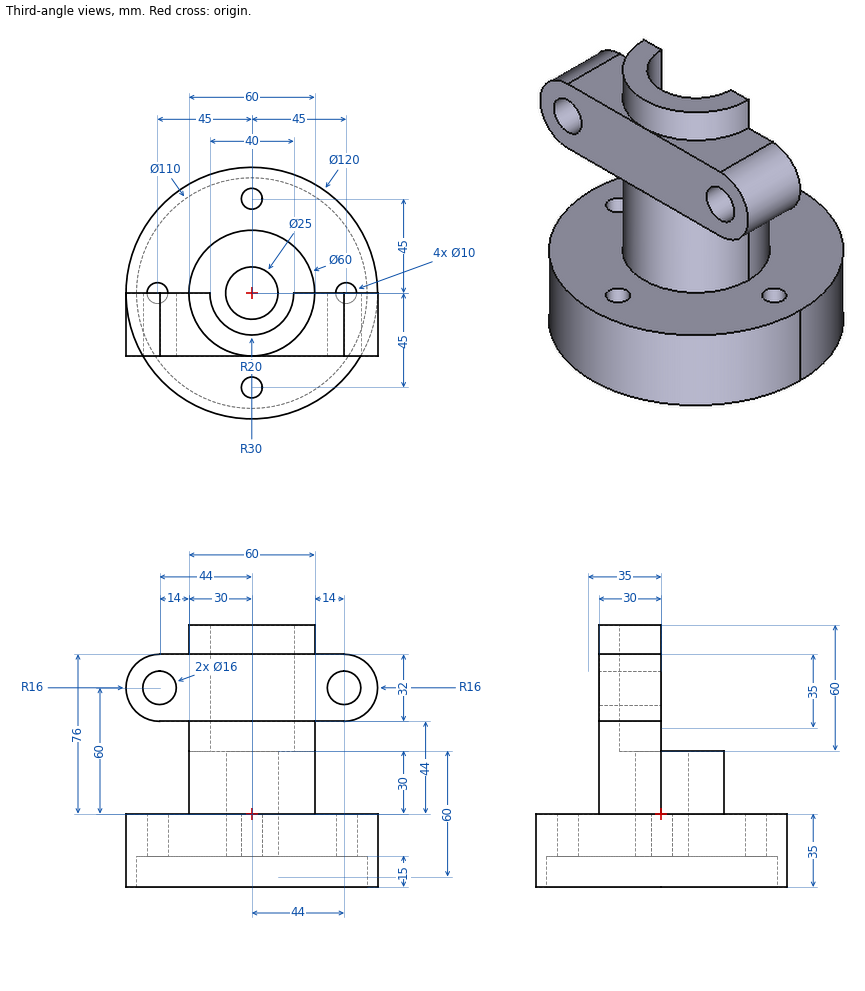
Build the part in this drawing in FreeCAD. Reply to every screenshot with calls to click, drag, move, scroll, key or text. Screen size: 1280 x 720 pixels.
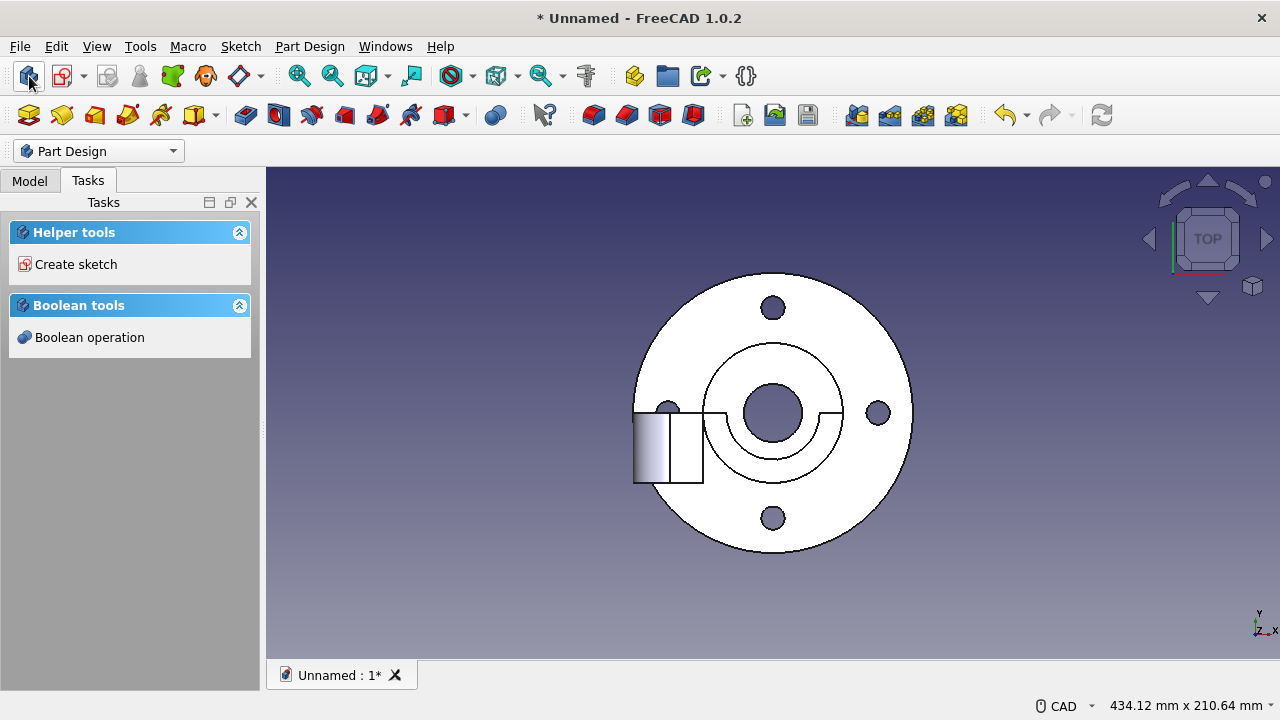
click(306, 619)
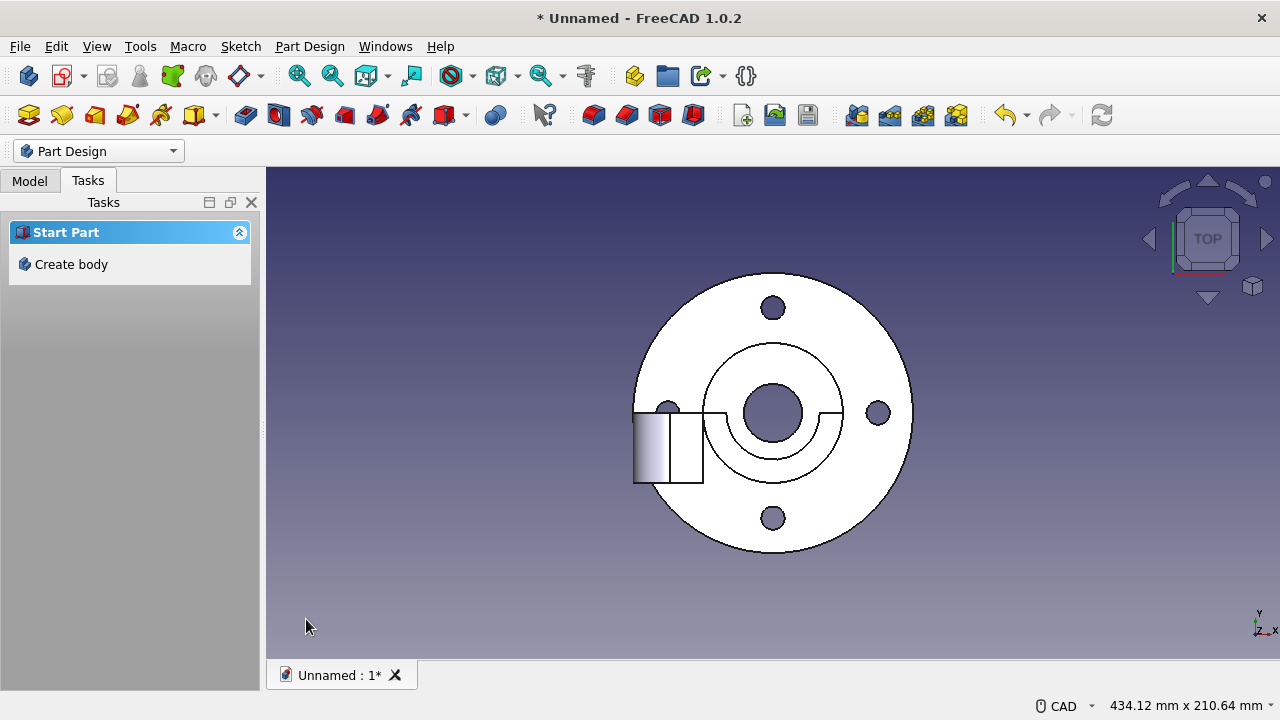
click(62, 76)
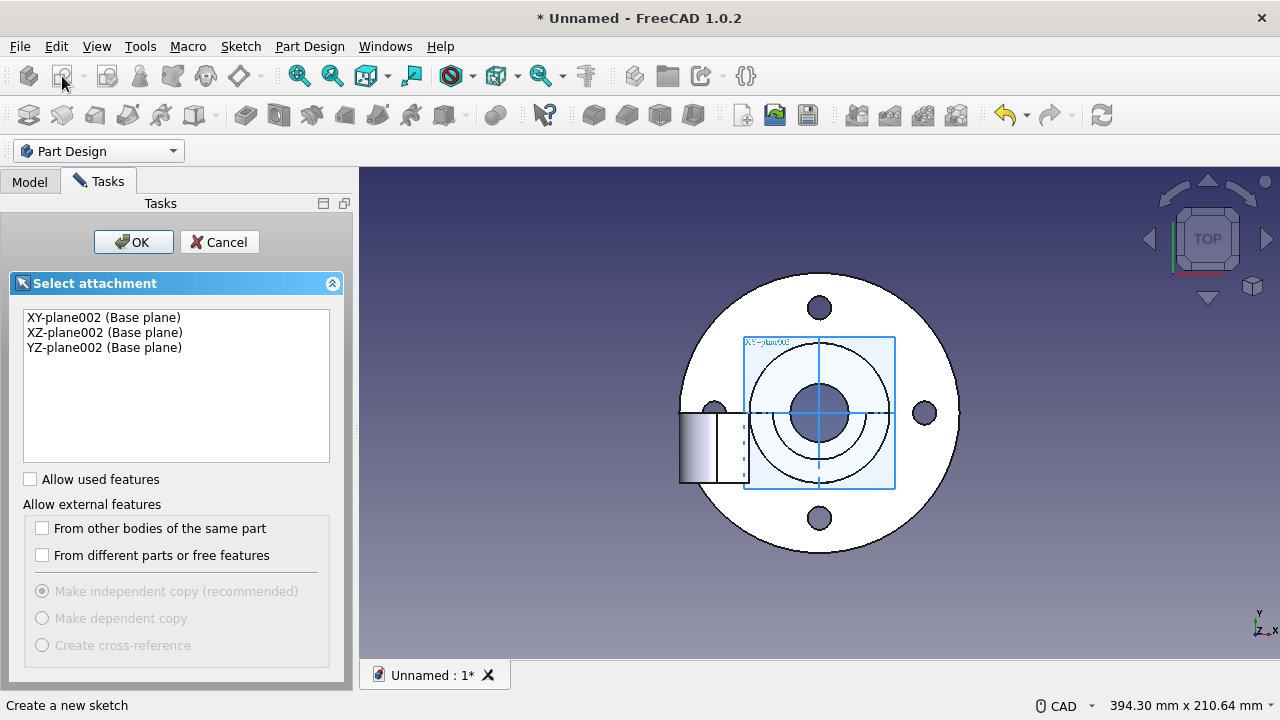
click(84, 332)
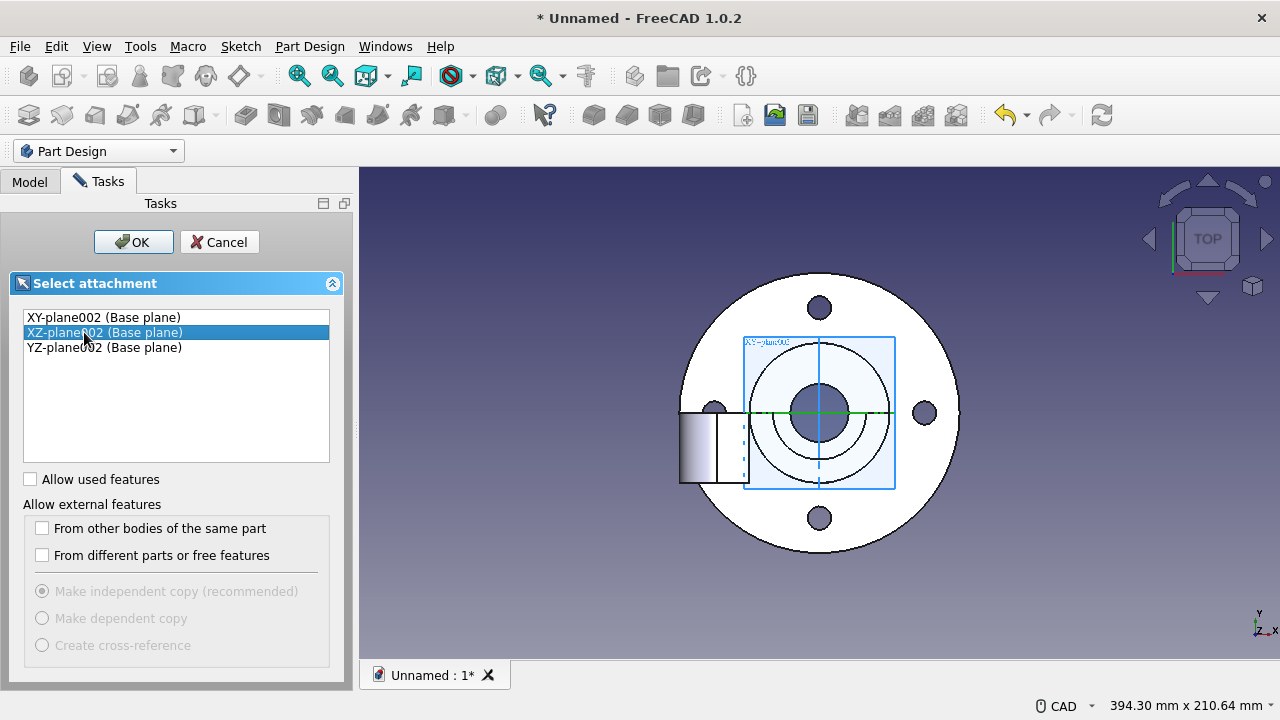
click(134, 242)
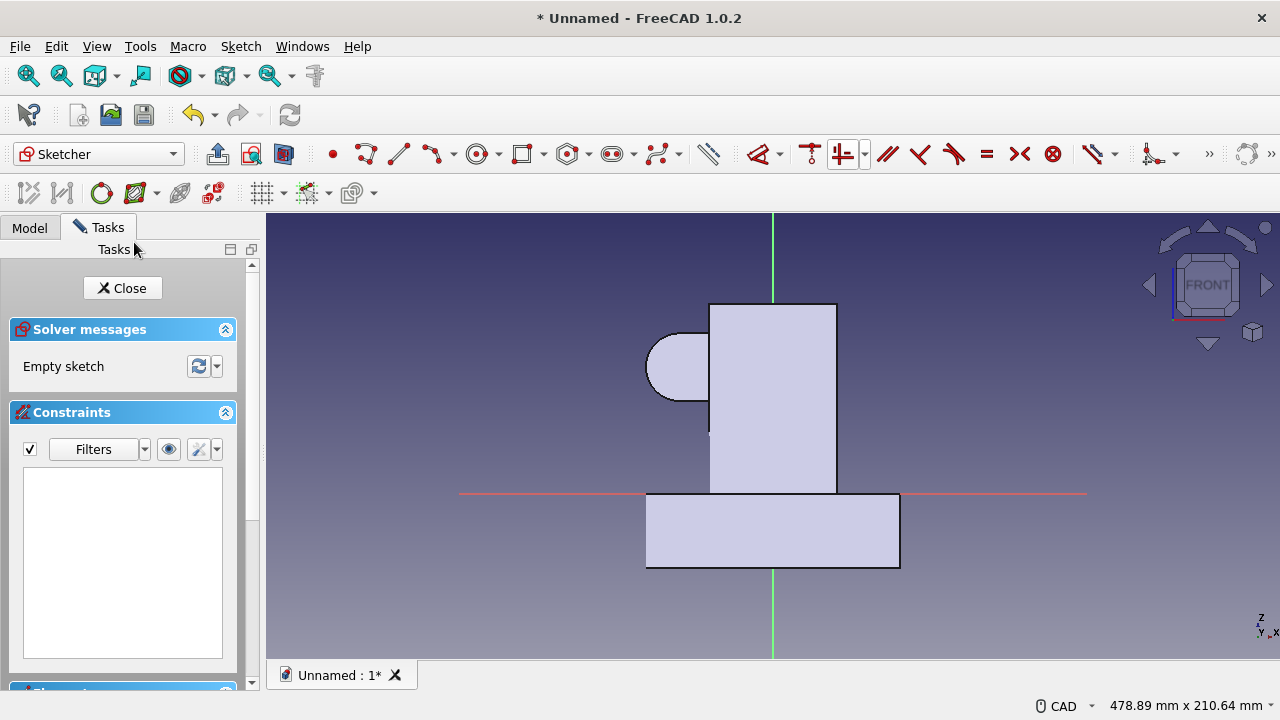
scroll(997, 387, up, 3)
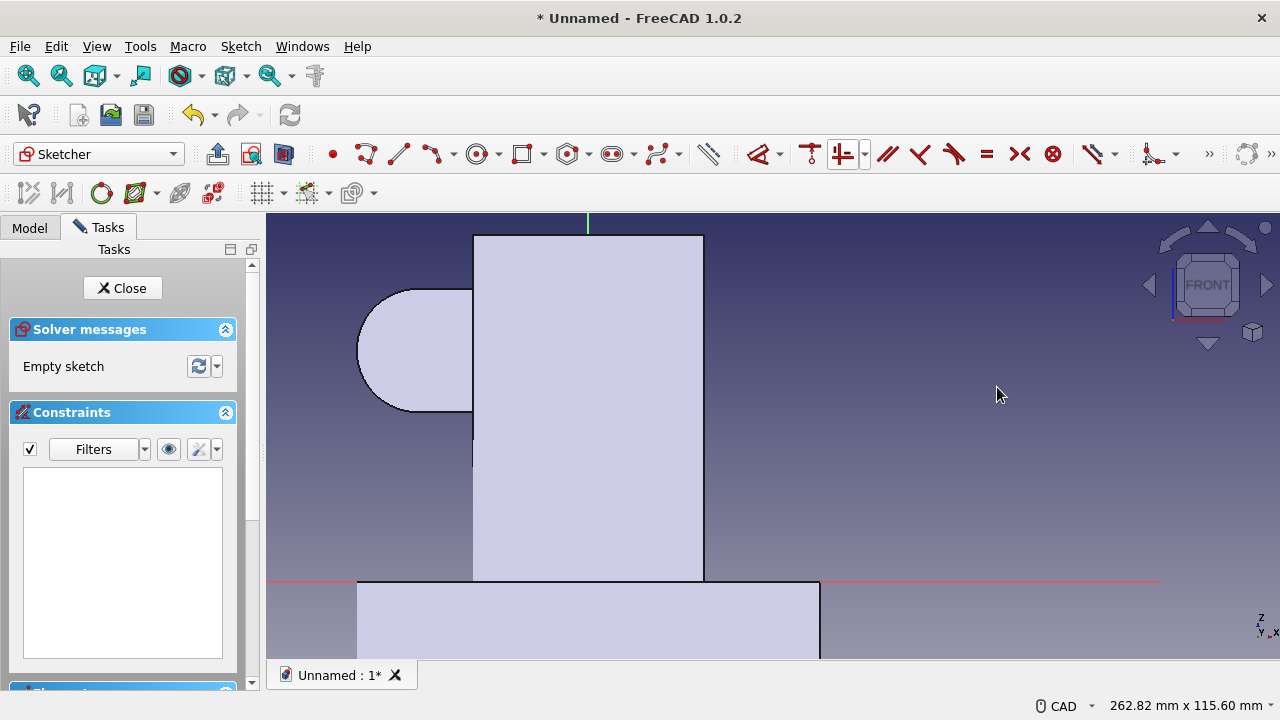
click(366, 154)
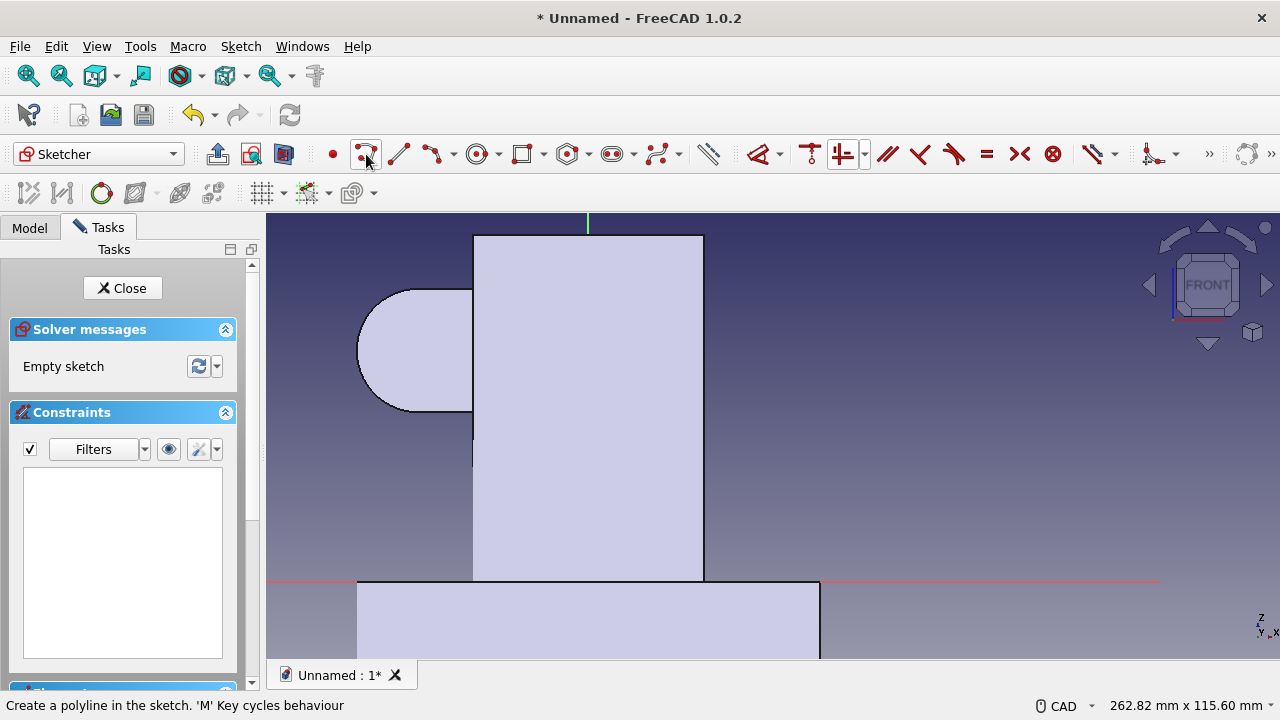
click(758, 412)
click(704, 412)
click(704, 289)
click(758, 289)
right_click(758, 289)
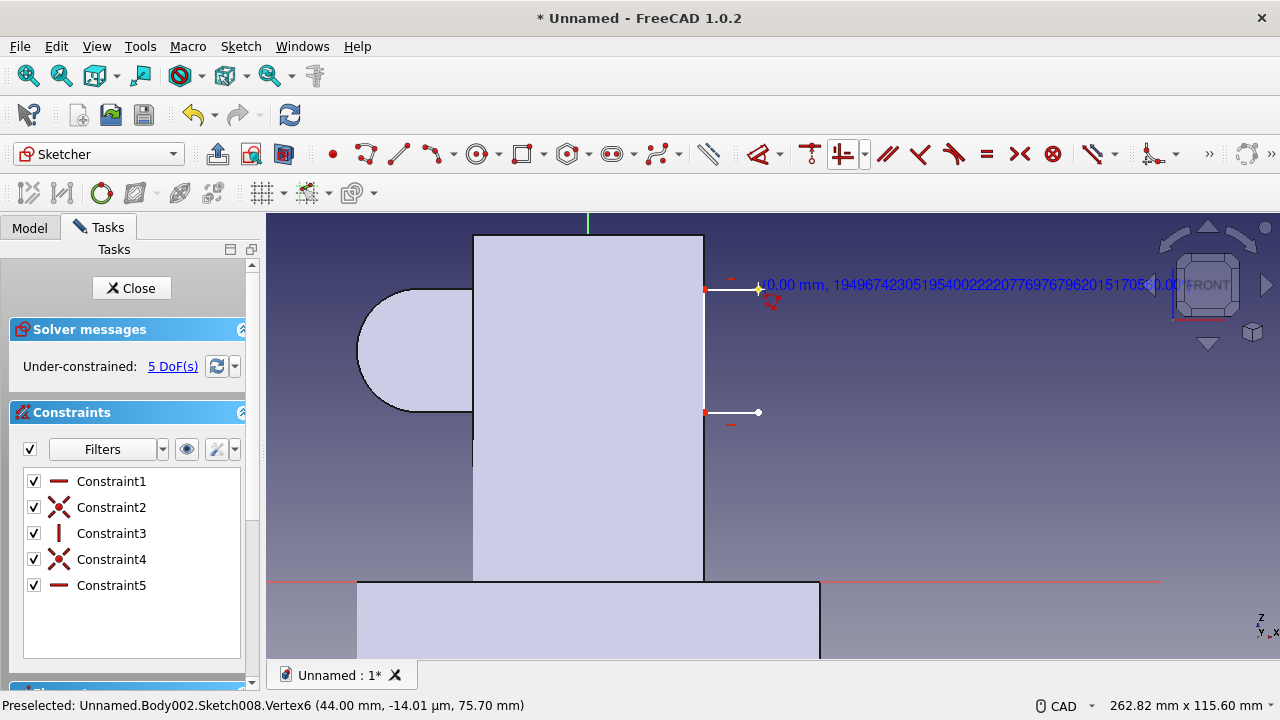
click(432, 154)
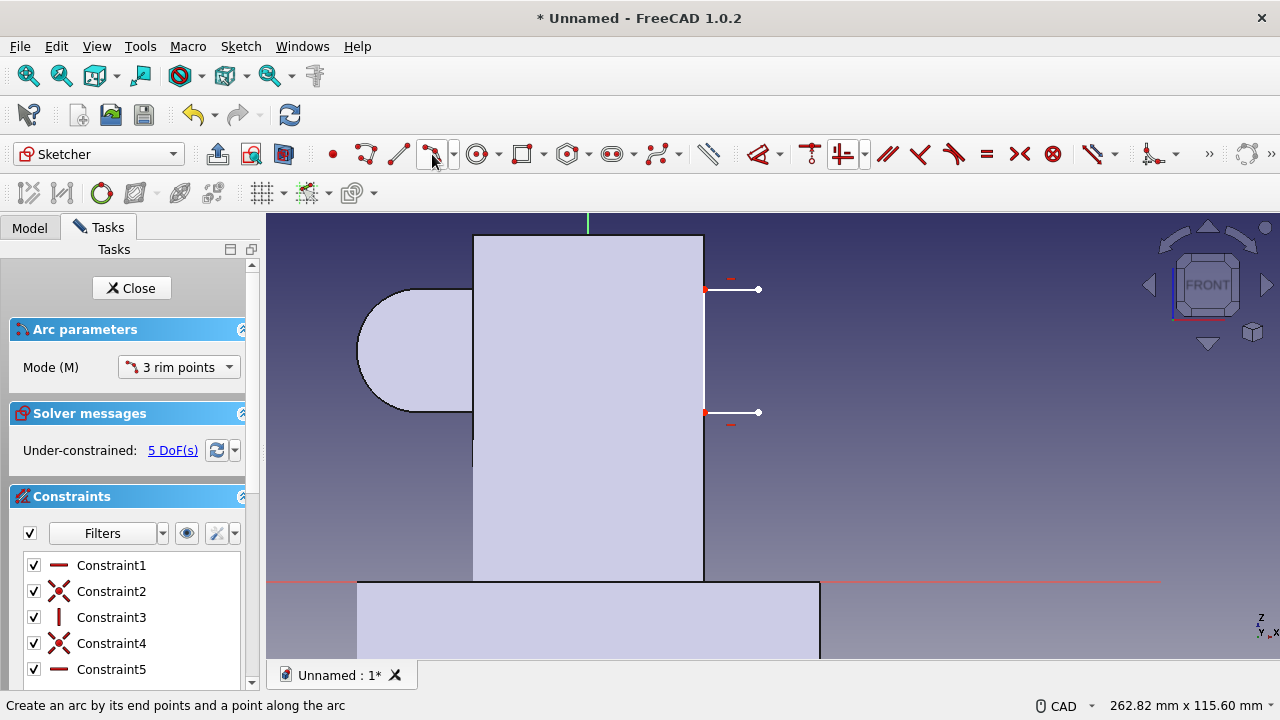
click(758, 290)
click(758, 413)
click(820, 351)
key(Escape)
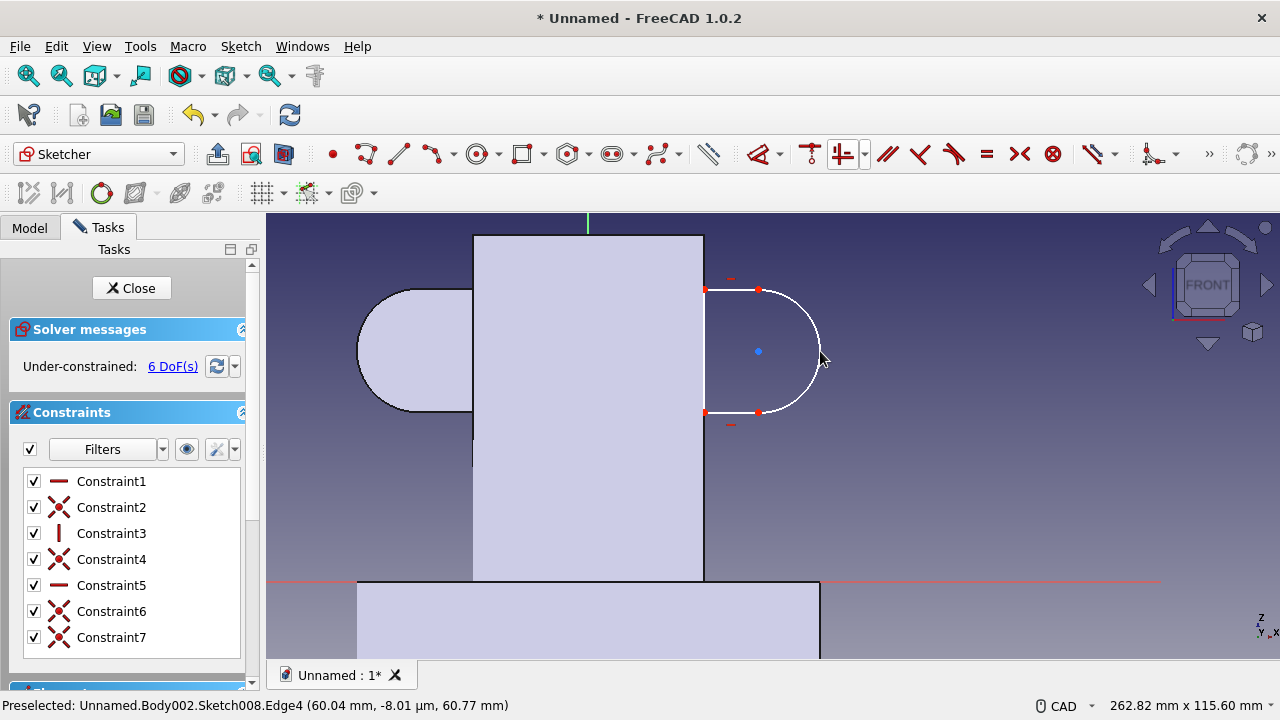
click(742, 413)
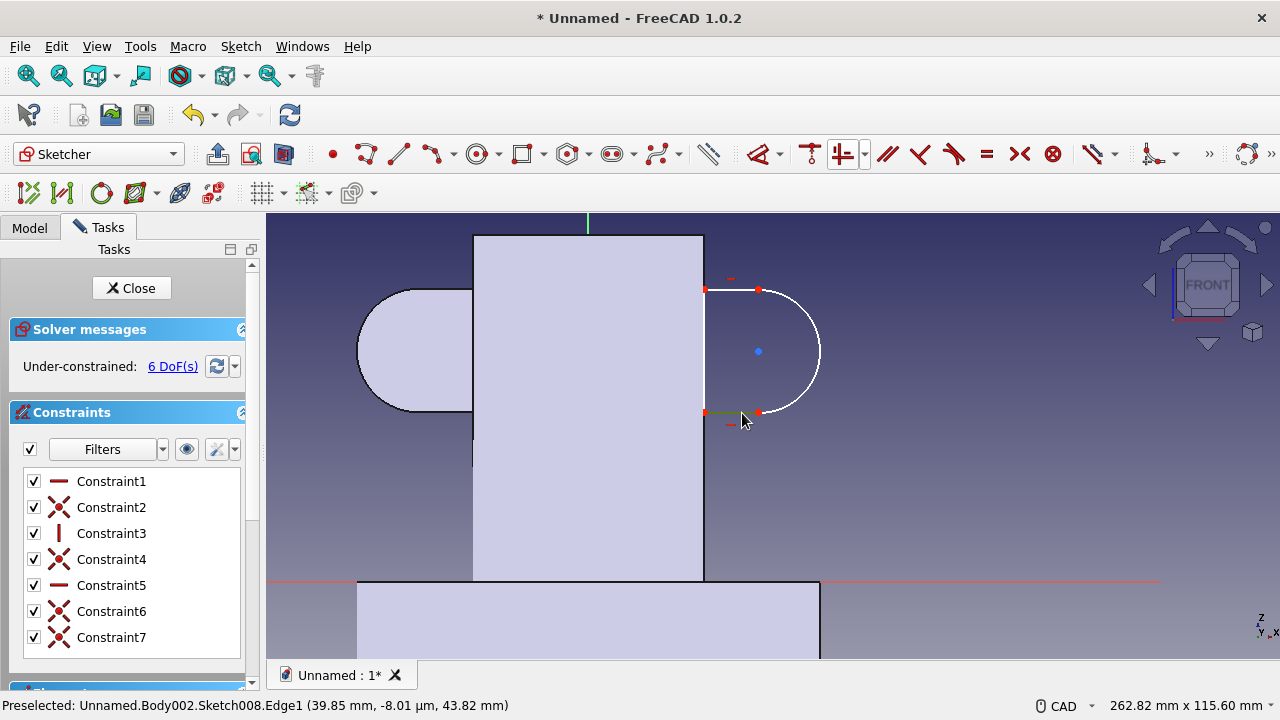
click(808, 388)